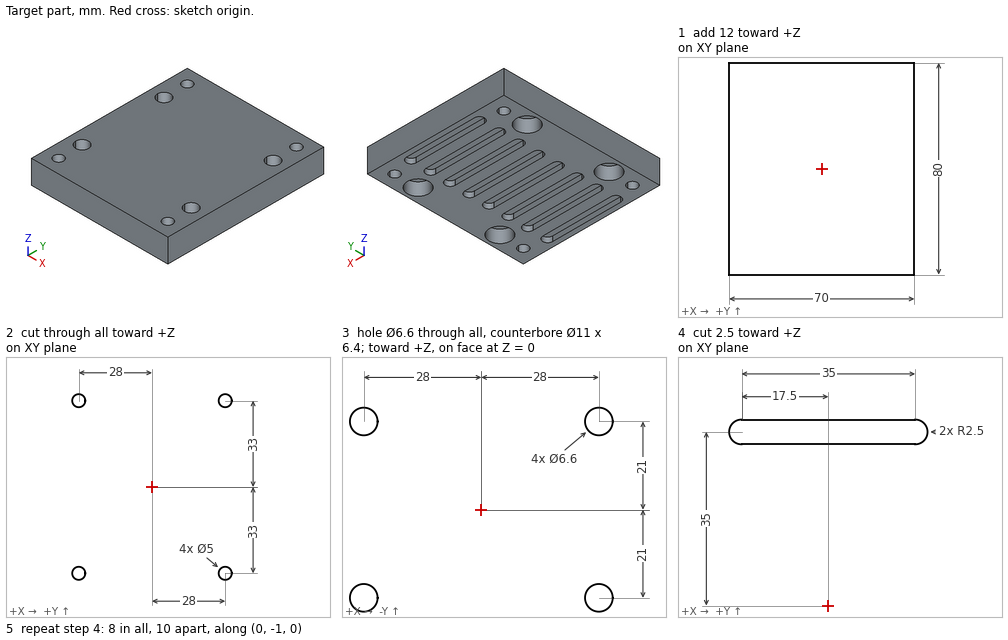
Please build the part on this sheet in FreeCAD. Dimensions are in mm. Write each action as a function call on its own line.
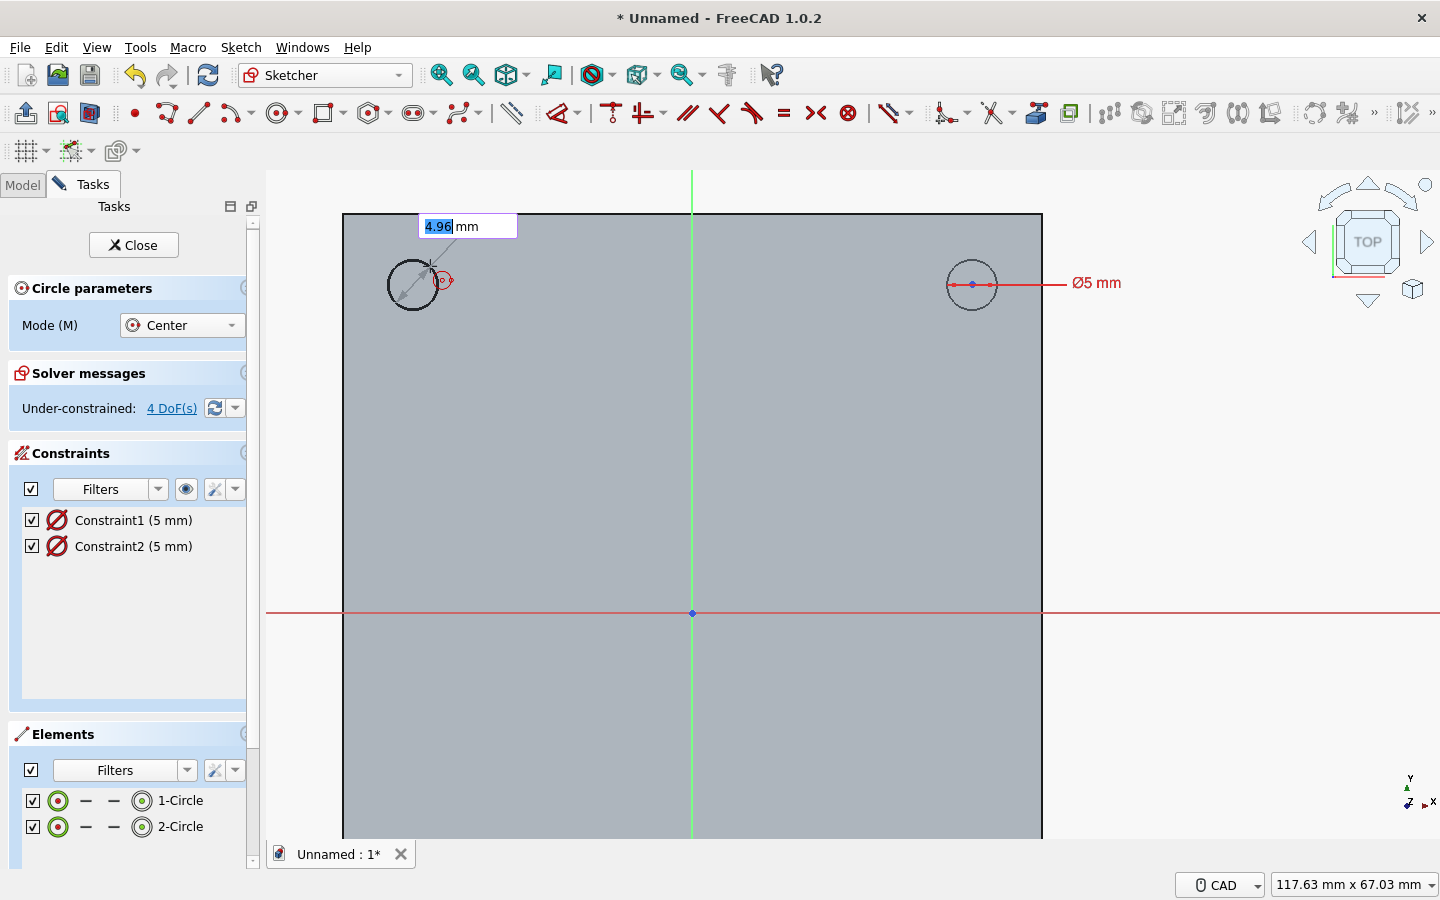
text(5)
key(Return)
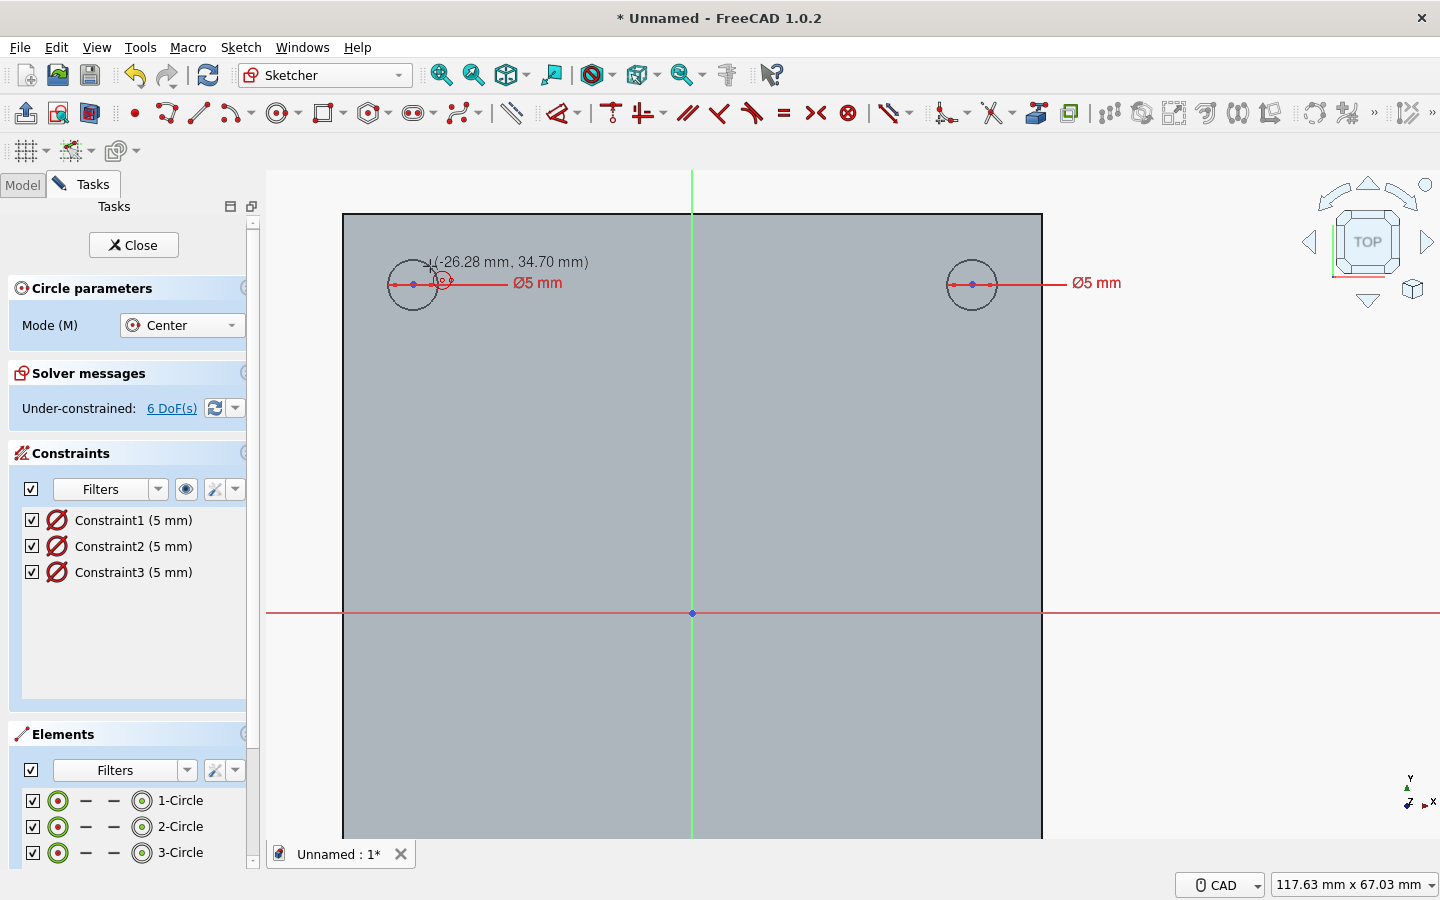
scroll(972, 283, down, 2)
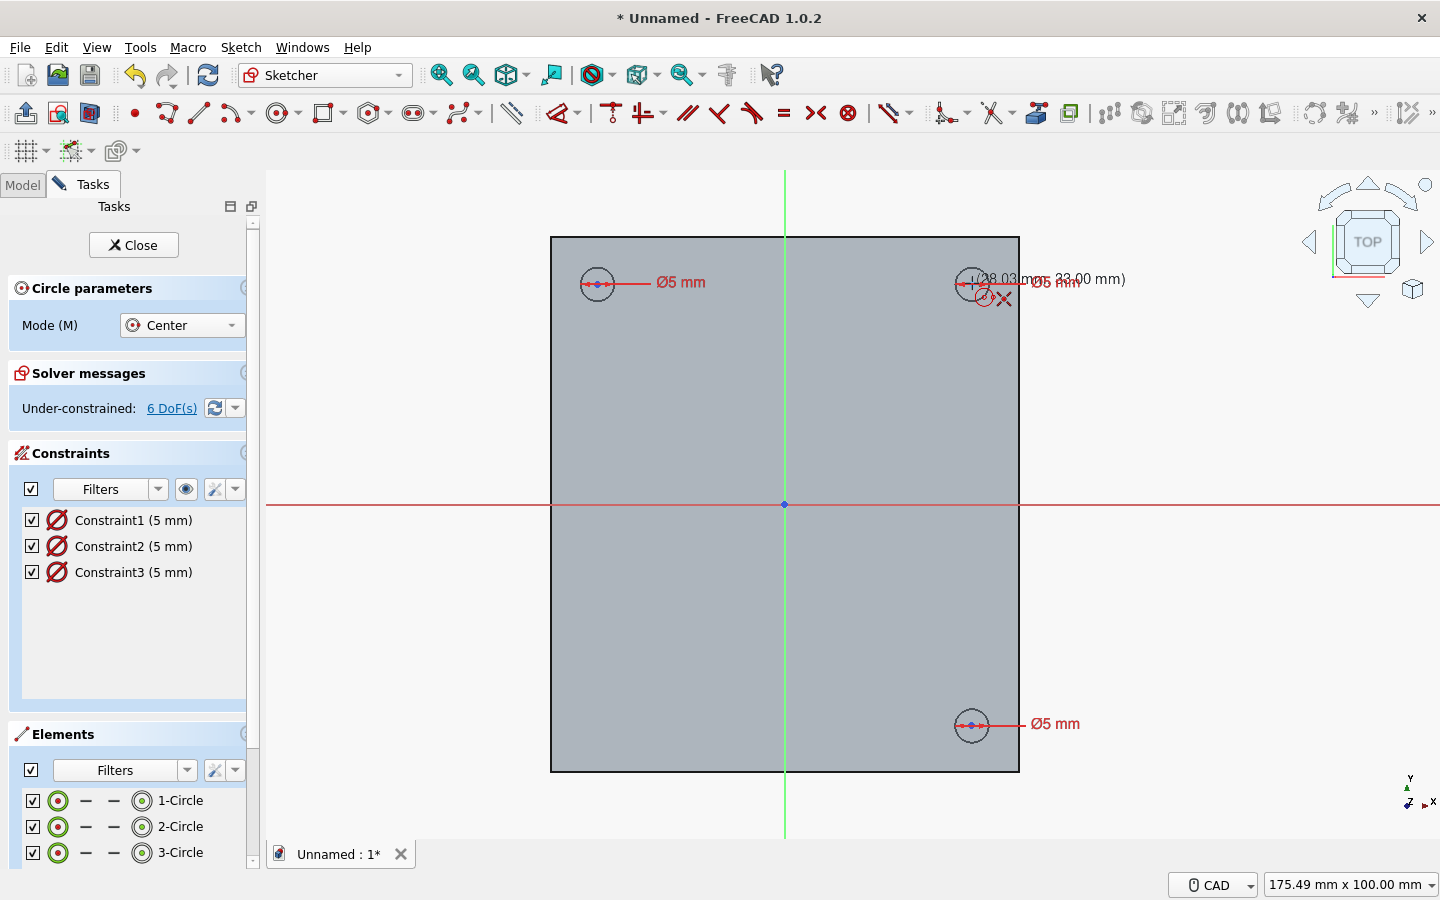
scroll(597, 725, up, 2)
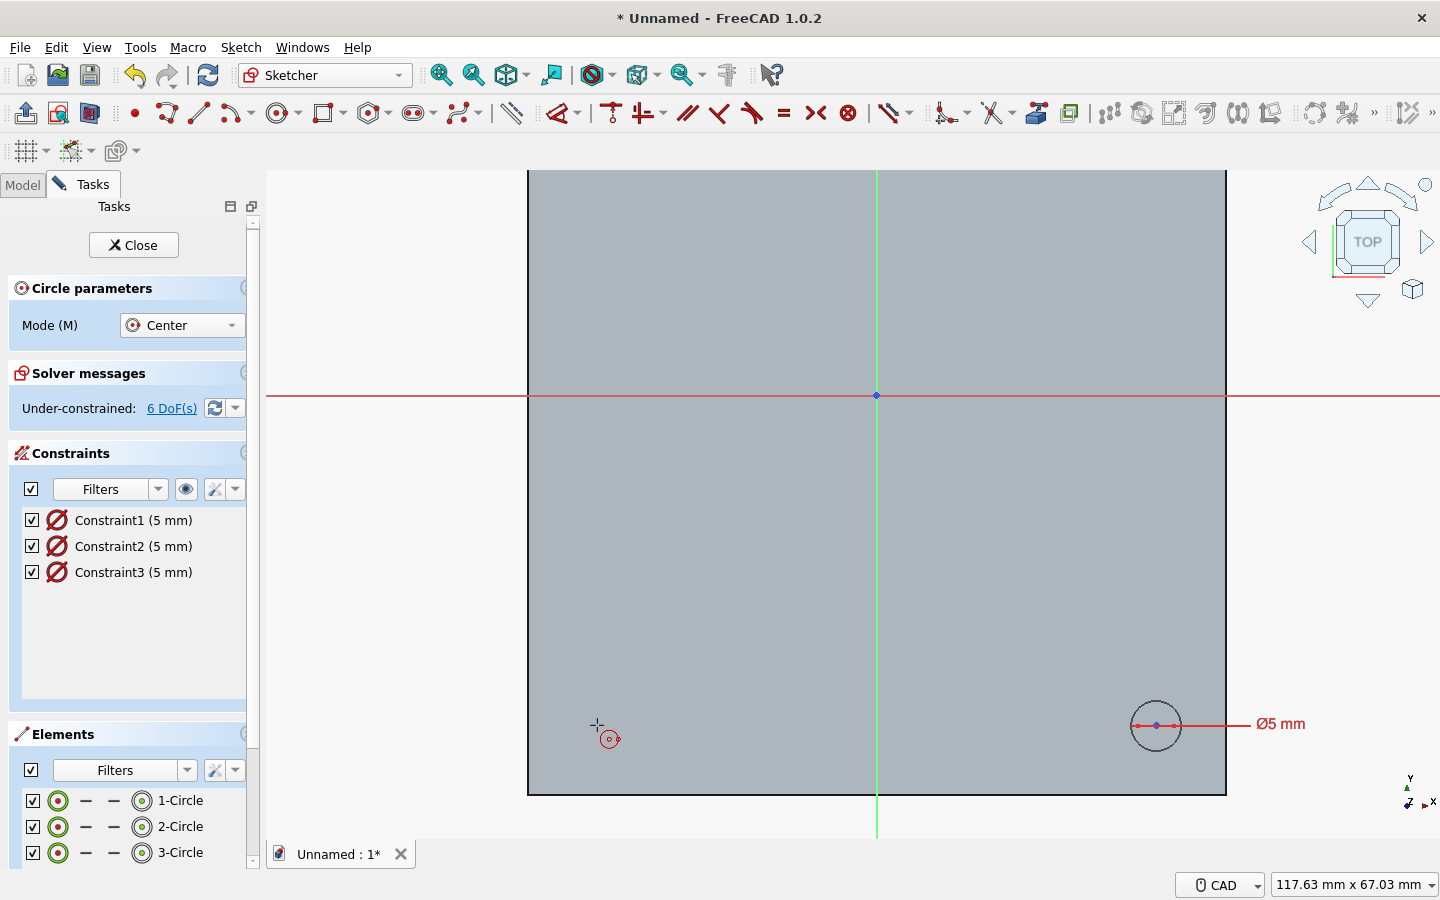
click(597, 725)
move(615, 707)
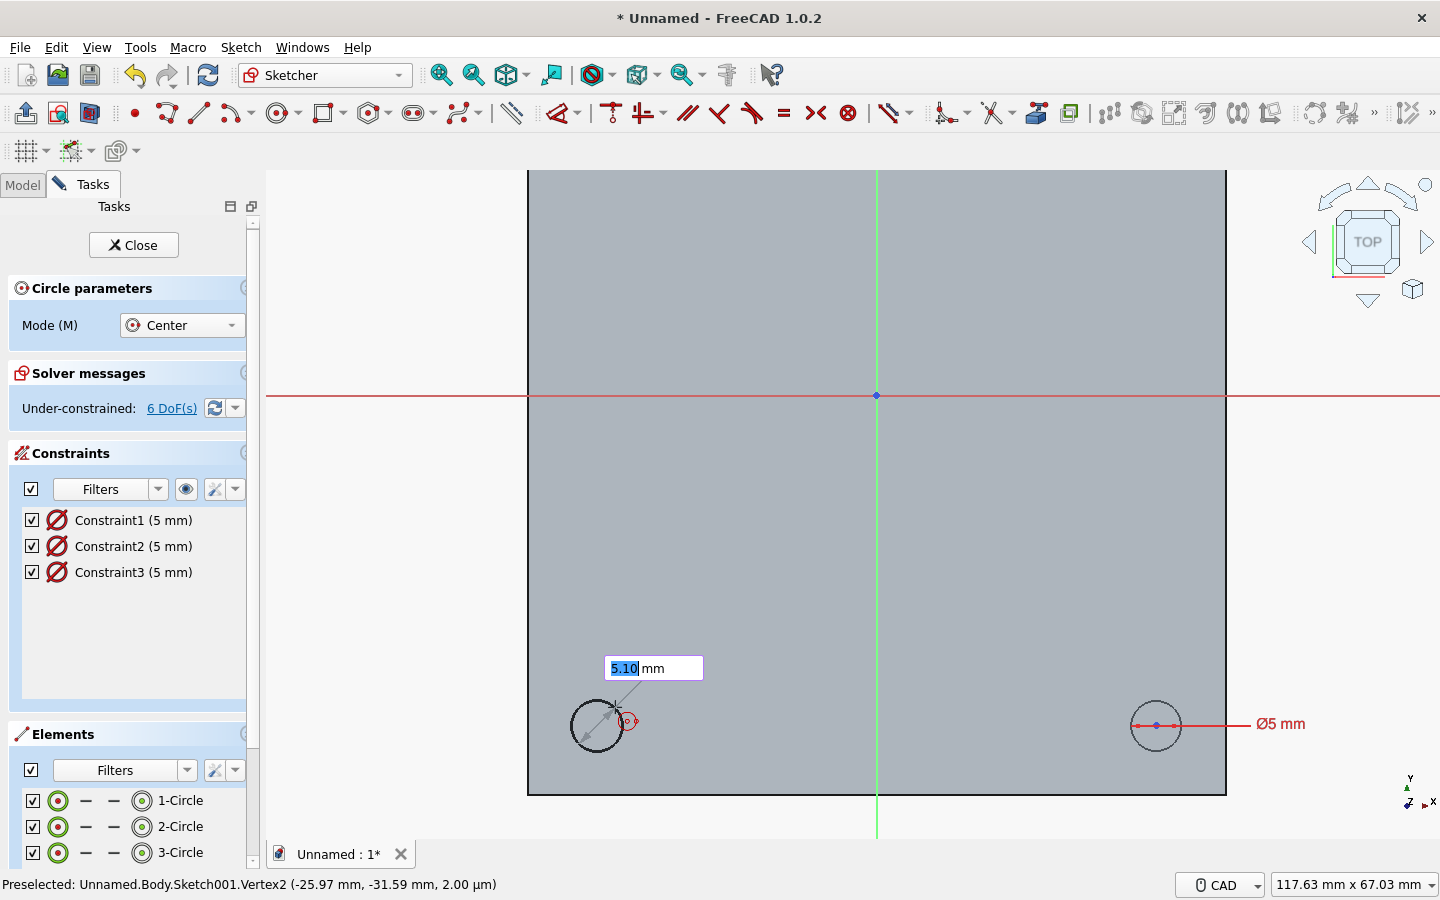
text(5)
key(Return)
key(Escape)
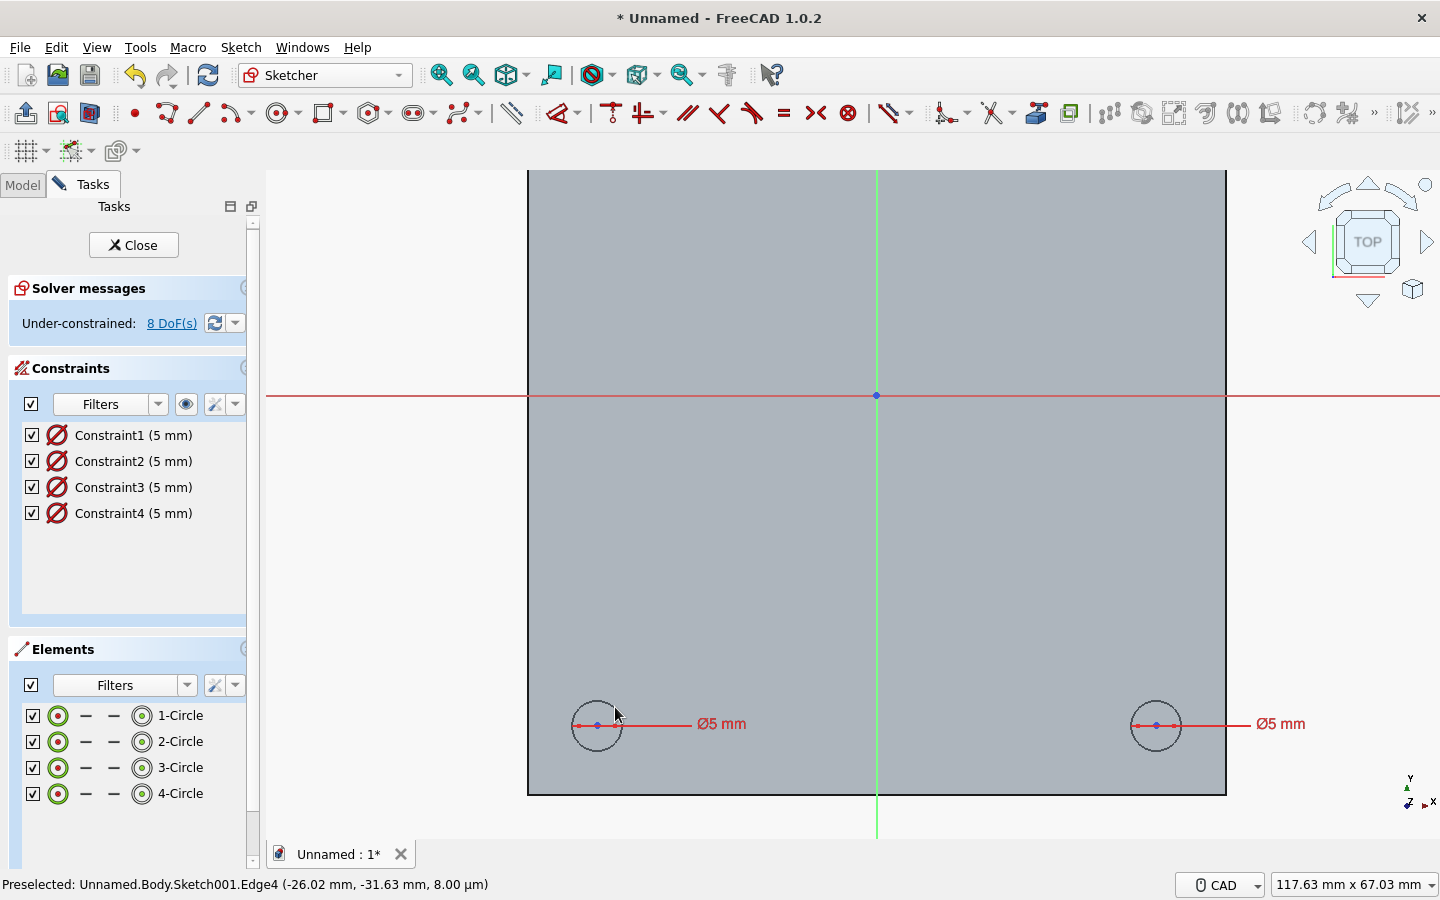
click(1156, 726)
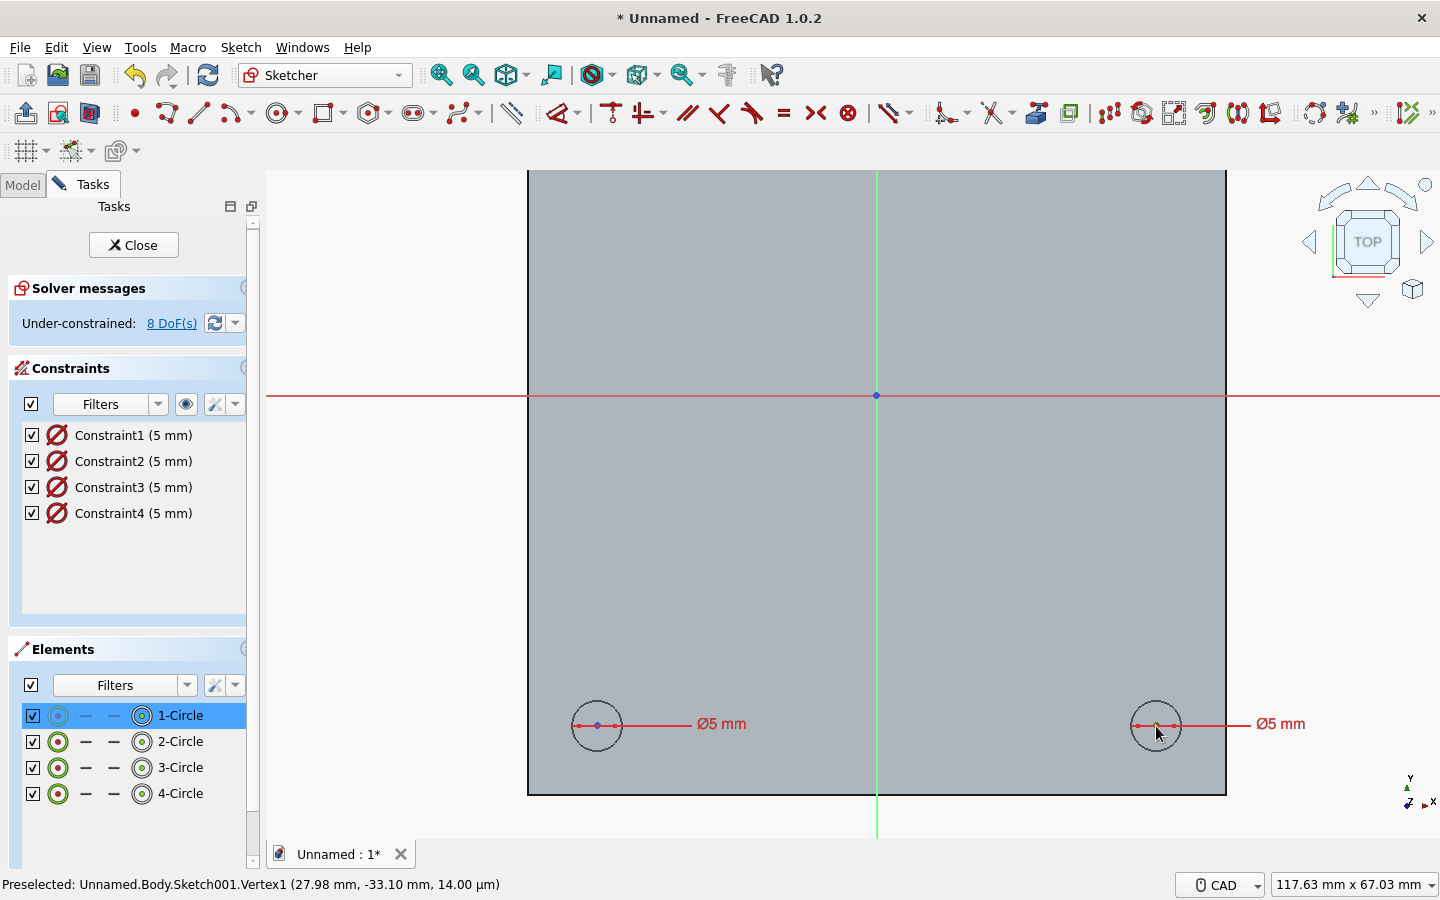
scroll(597, 726, down, 2)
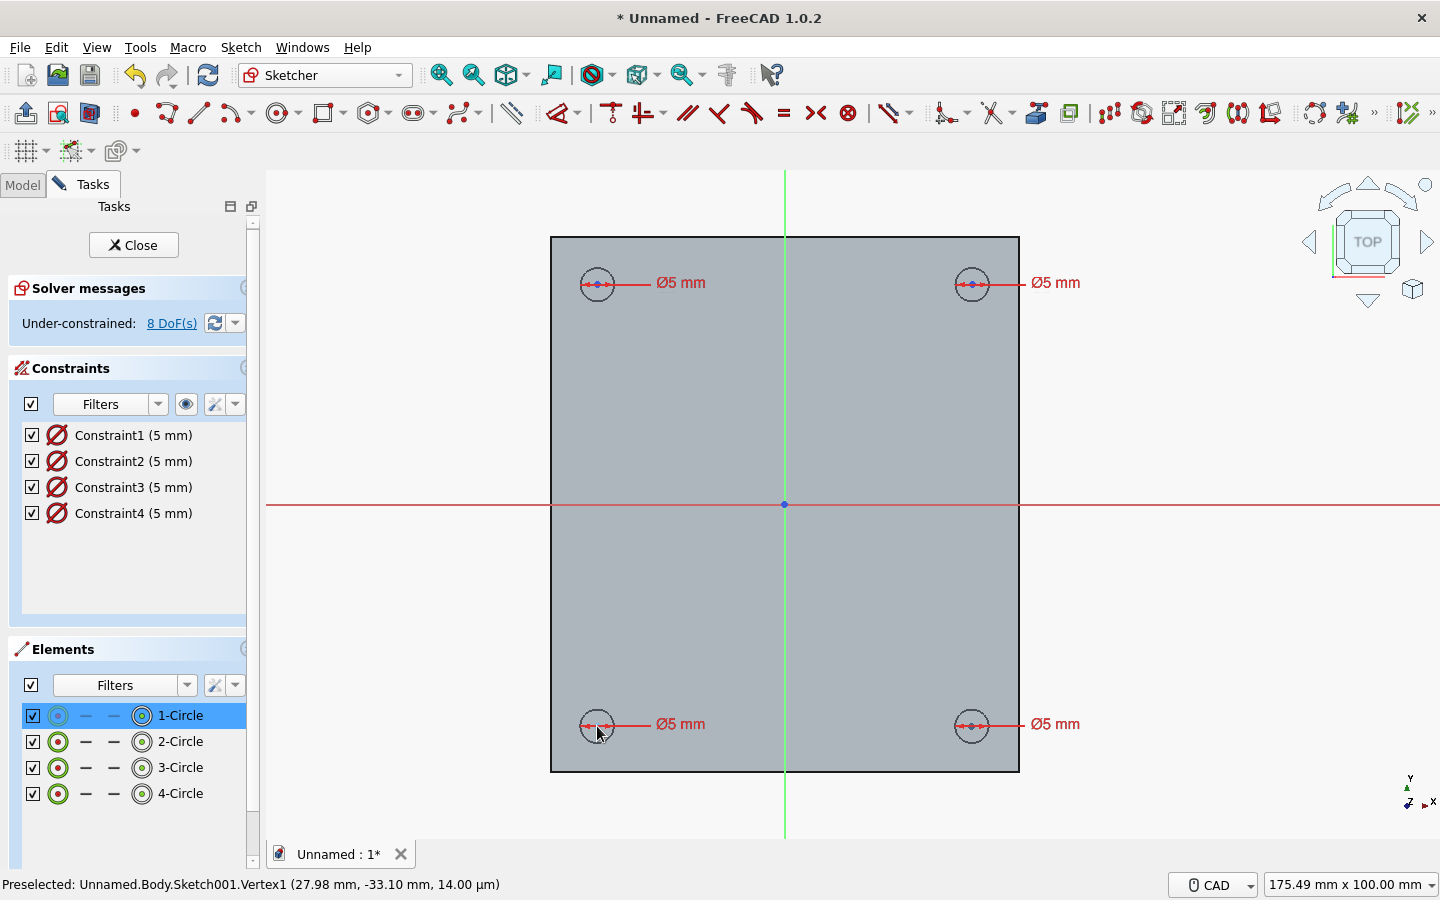
click(972, 285)